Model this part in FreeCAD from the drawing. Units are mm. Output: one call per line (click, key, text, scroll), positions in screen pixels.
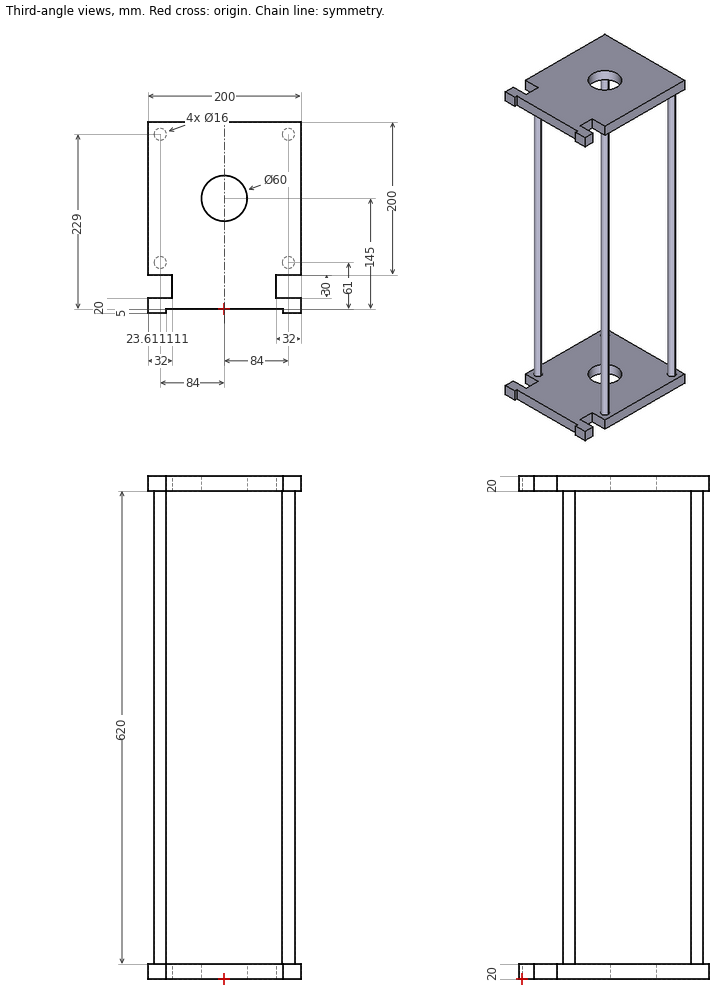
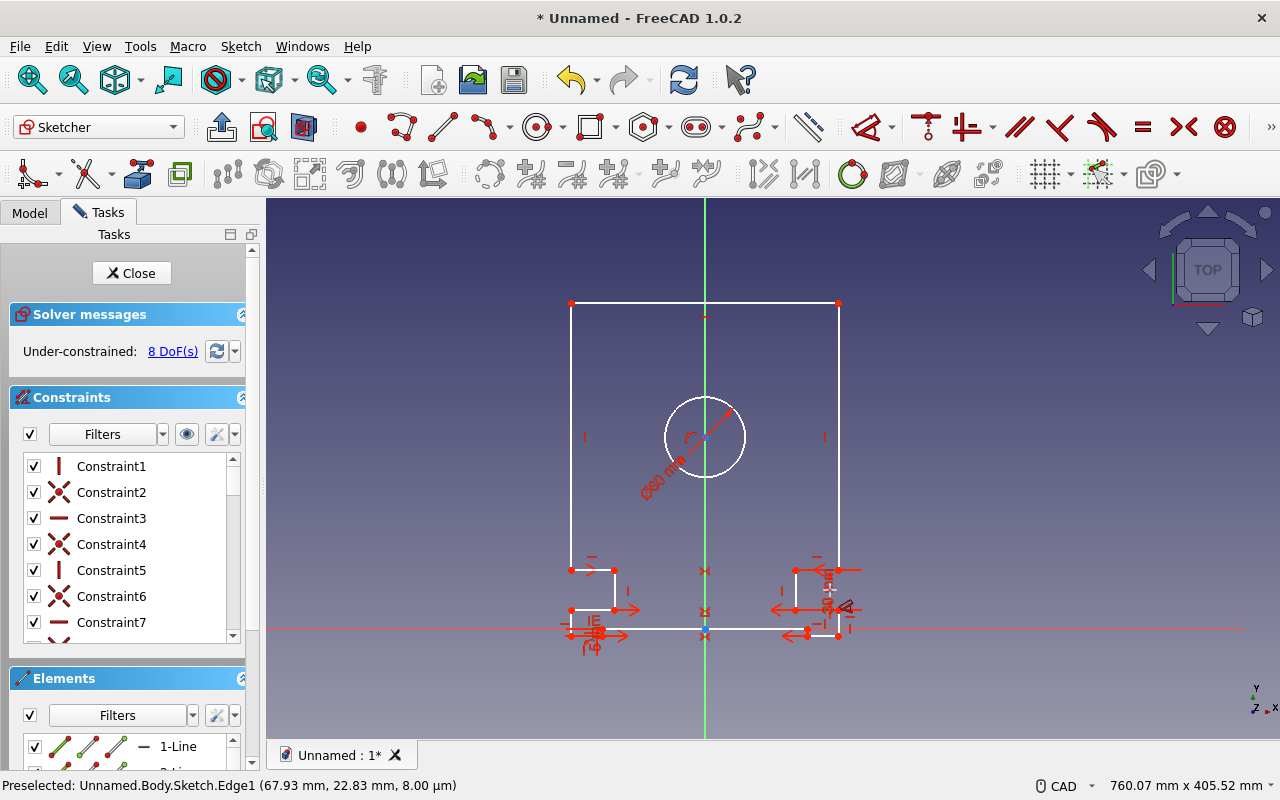
click(809, 570)
click(817, 536)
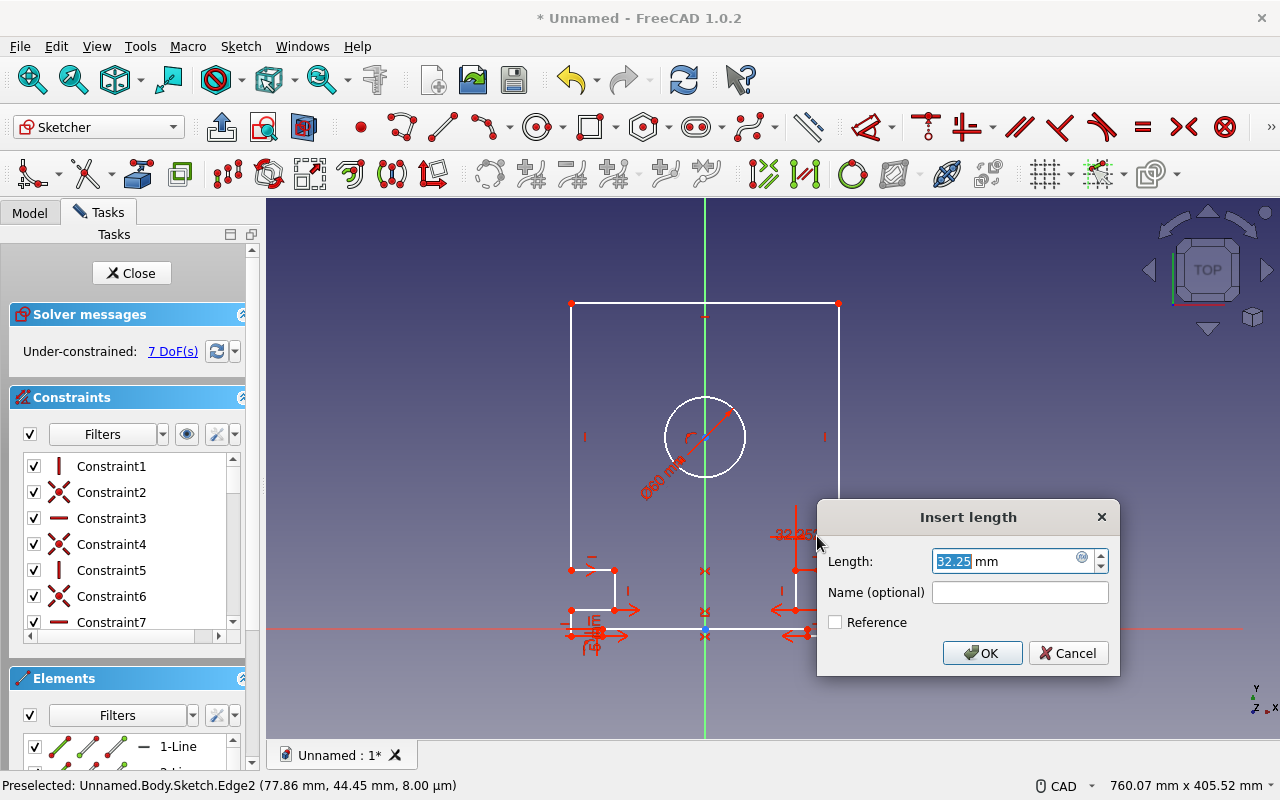
text(32)
key(Return)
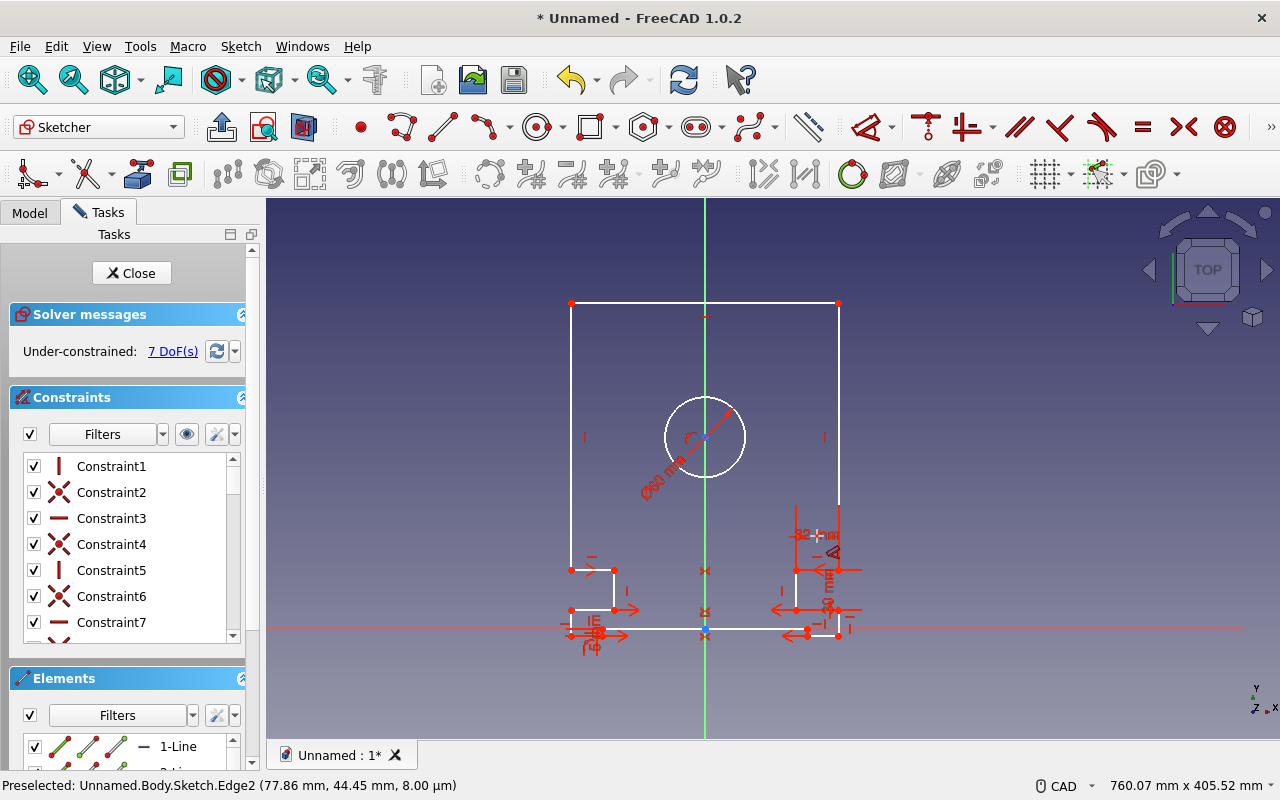
click(601, 610)
click(593, 668)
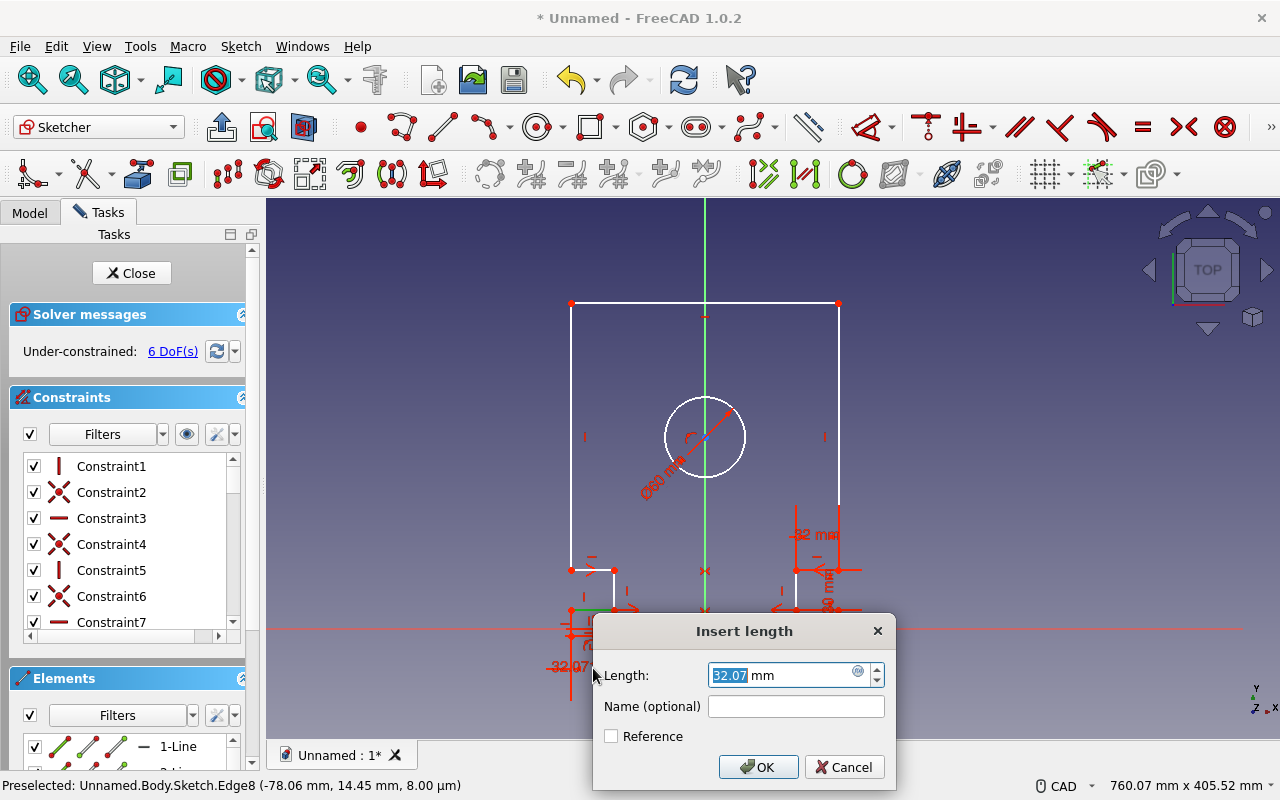
text(32)
key(Return)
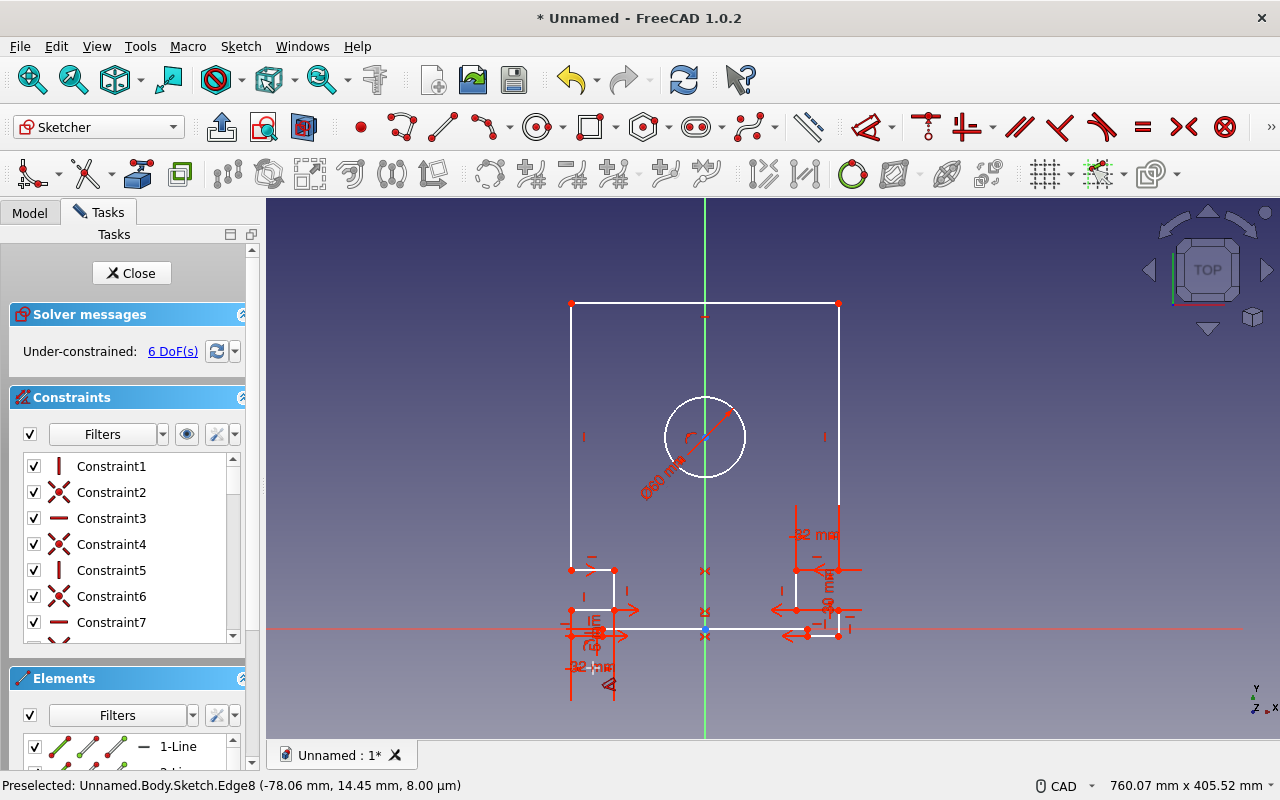
scroll(571, 626, up, 2)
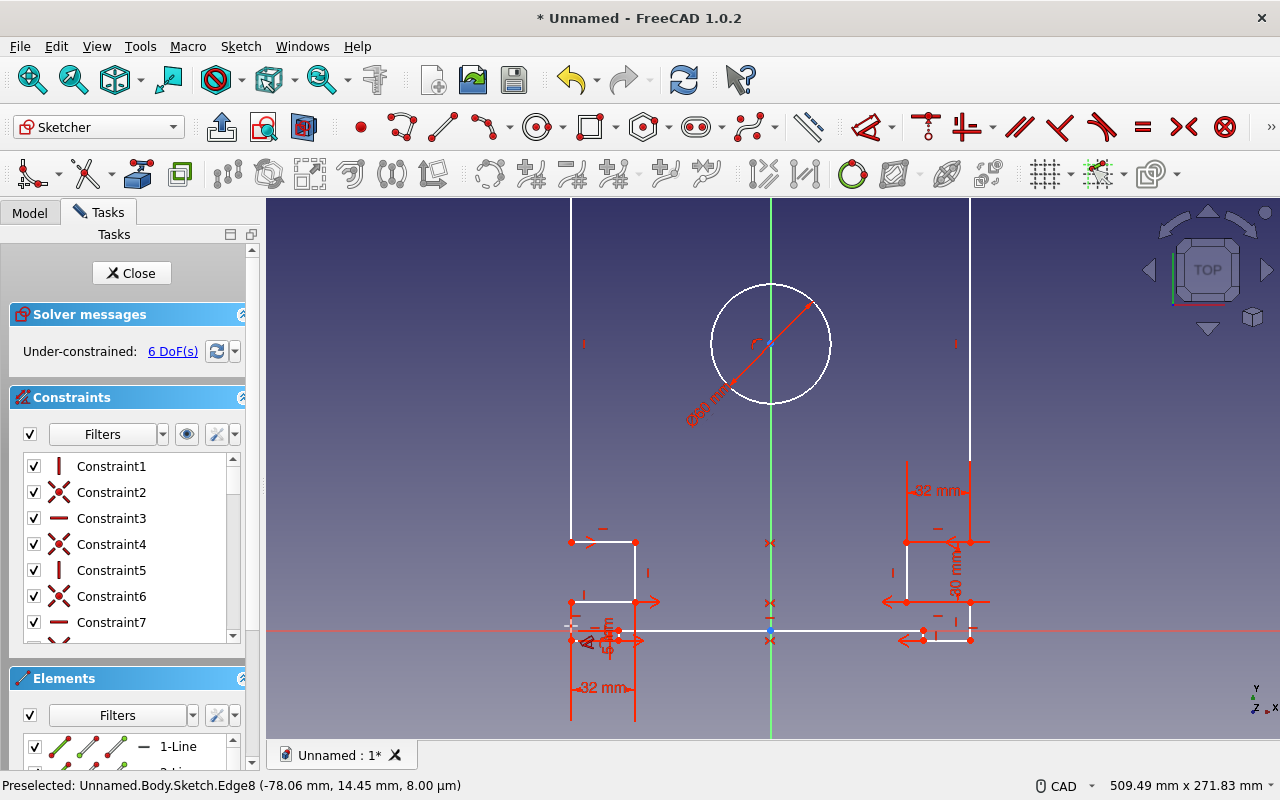
click(571, 625)
click(537, 612)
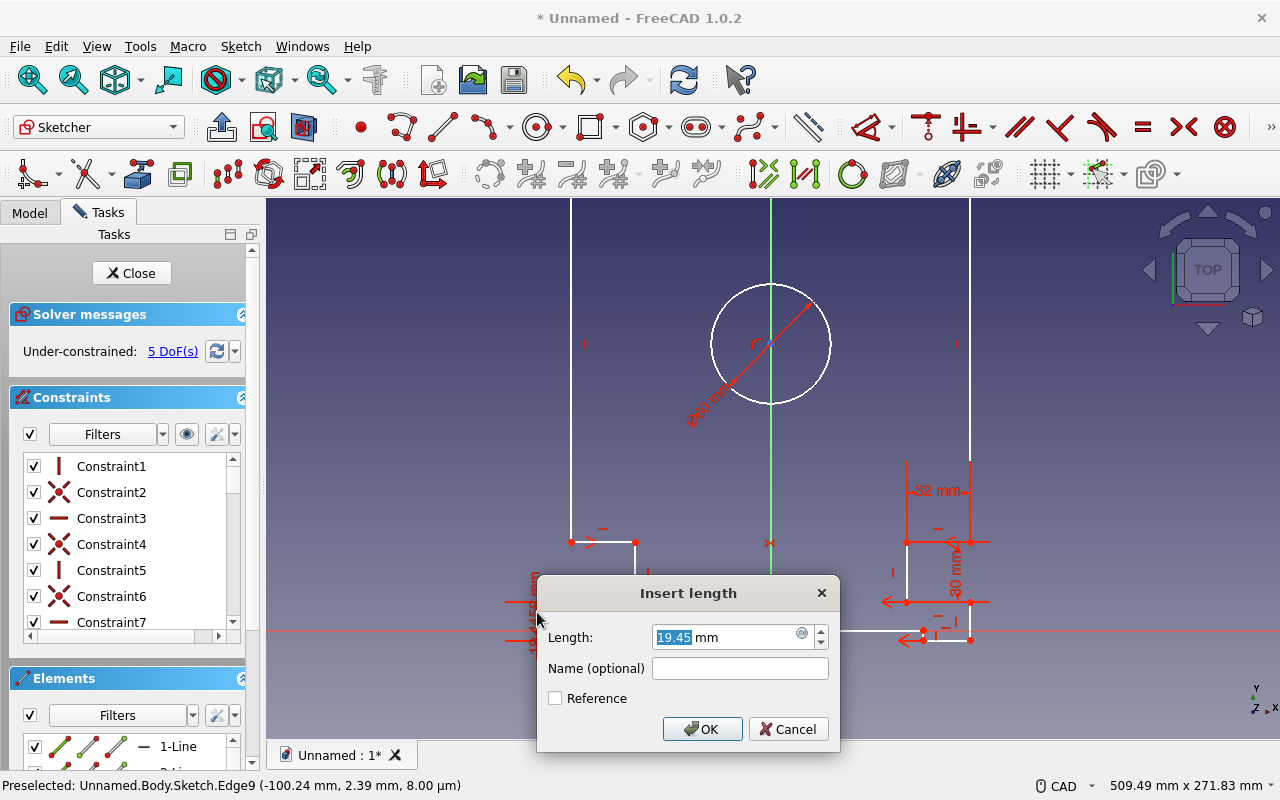
text(20)
key(Return)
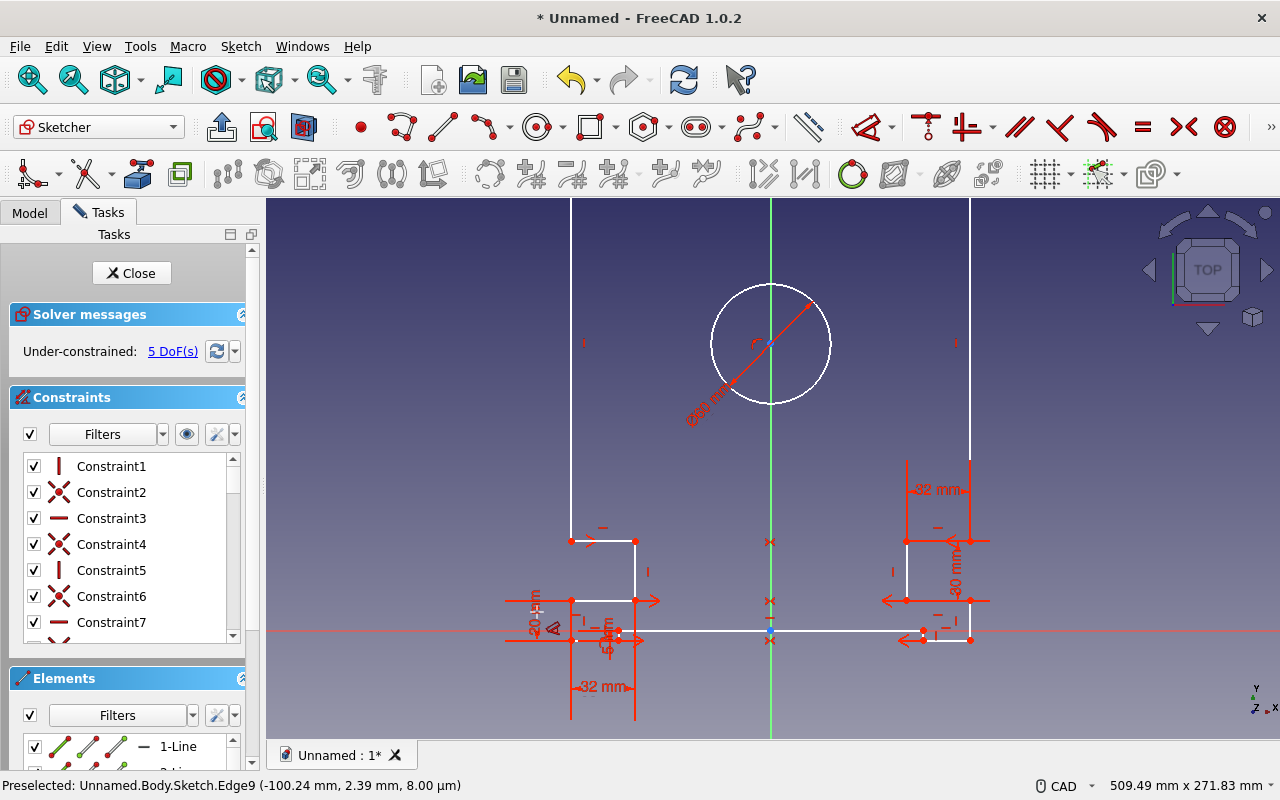
click(951, 601)
click(938, 659)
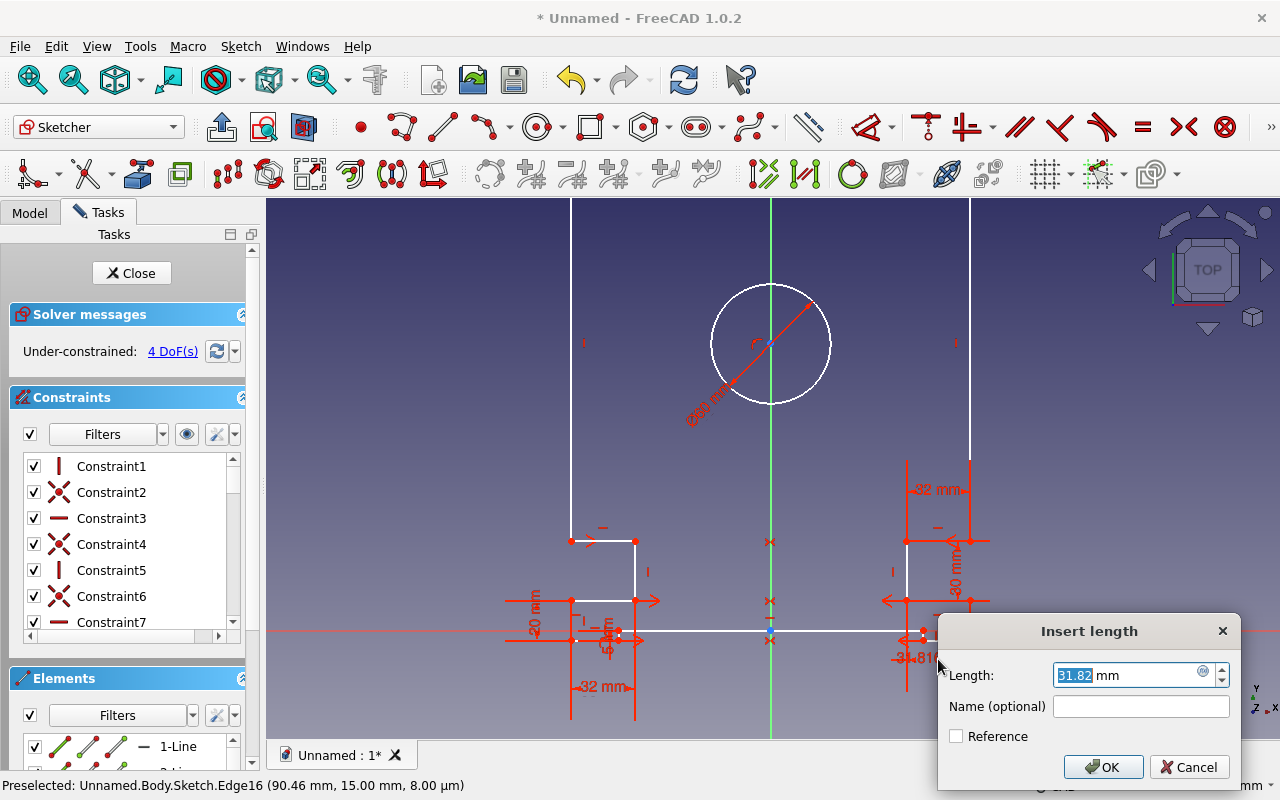
text(32)
key(Return)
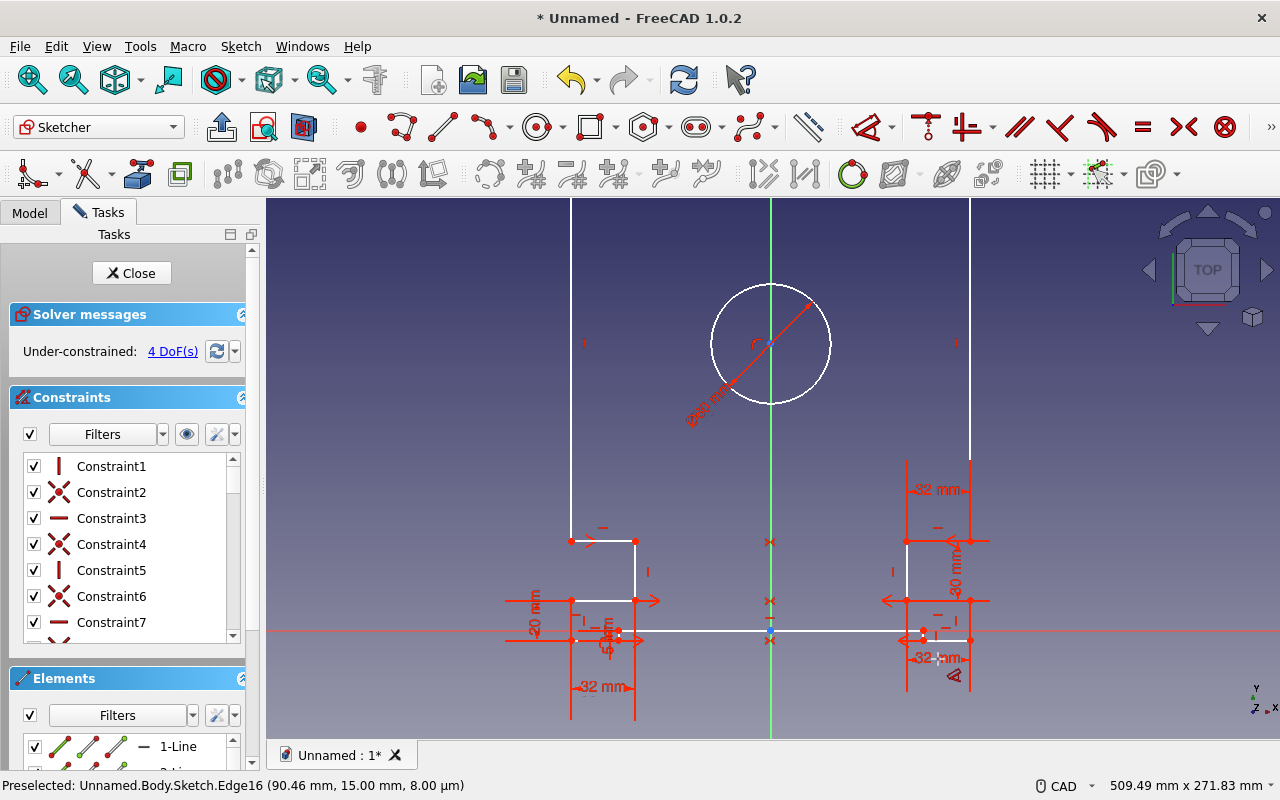
click(970, 422)
click(1004, 384)